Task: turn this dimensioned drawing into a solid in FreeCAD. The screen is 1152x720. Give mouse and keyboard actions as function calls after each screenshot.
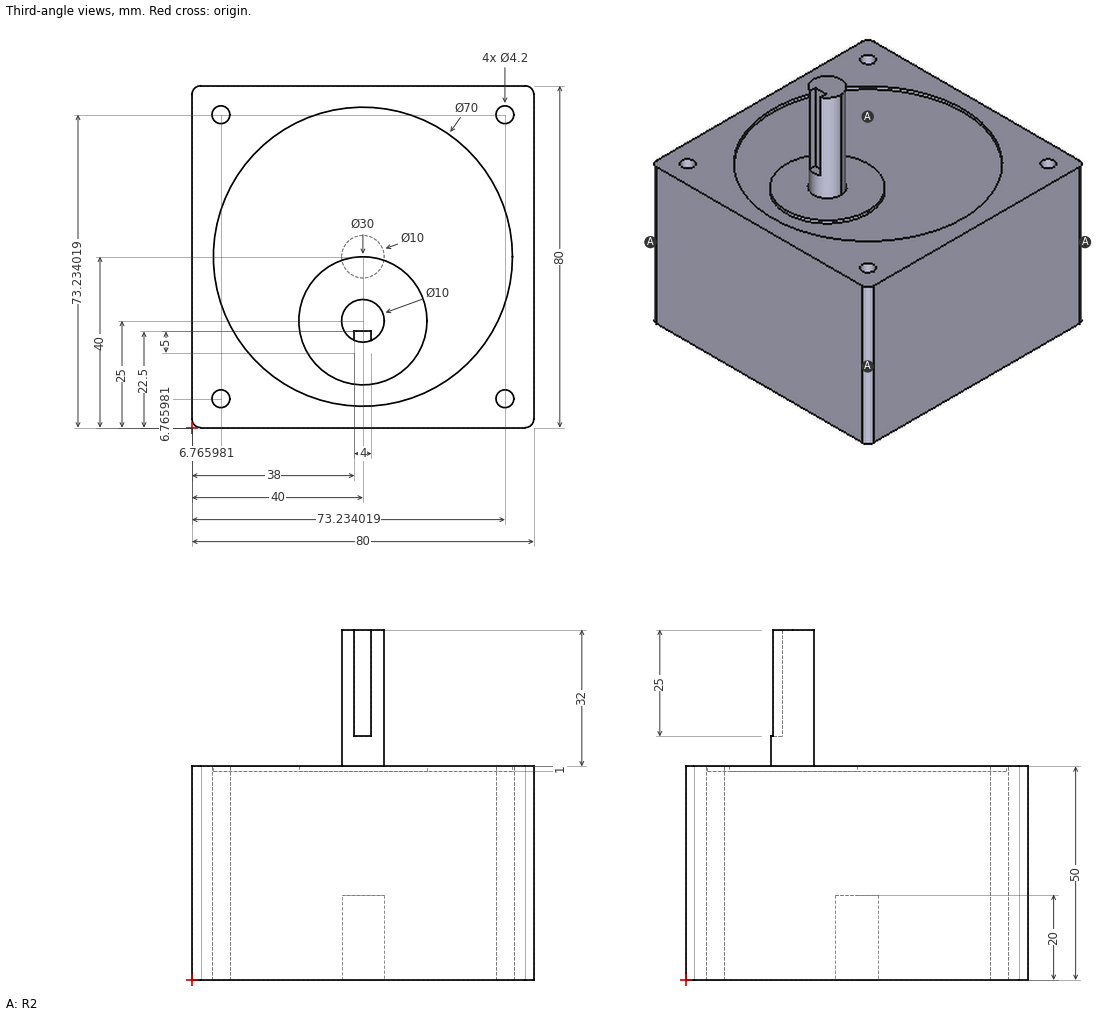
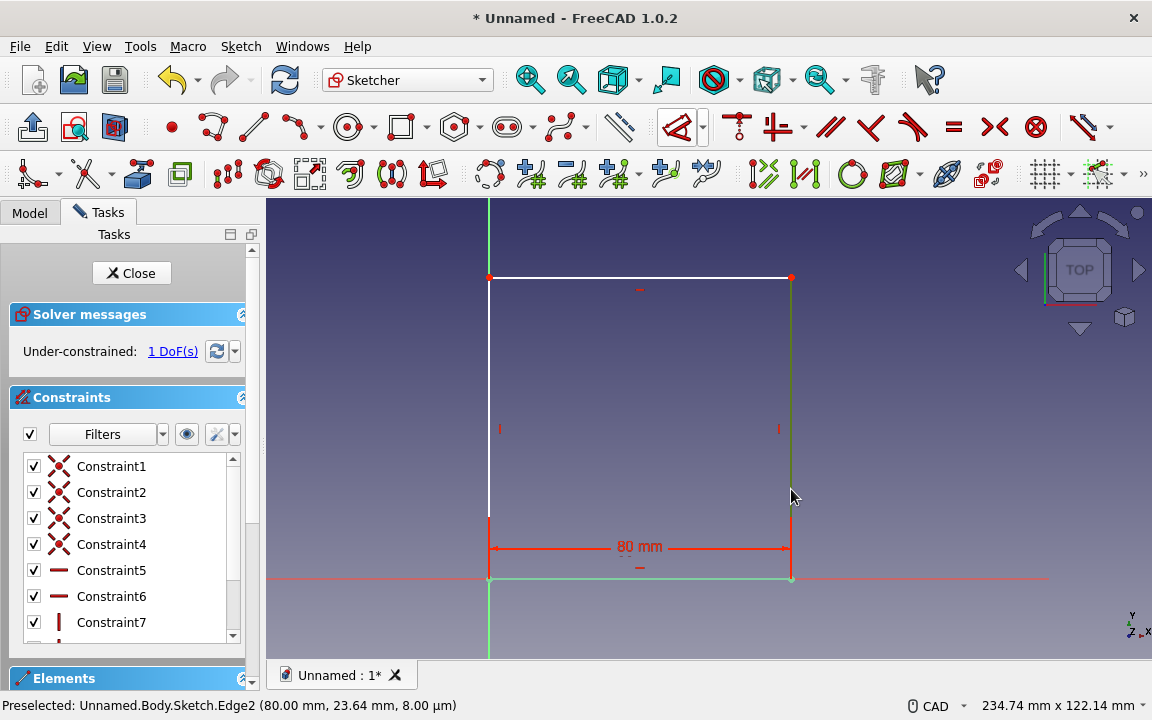
click(702, 128)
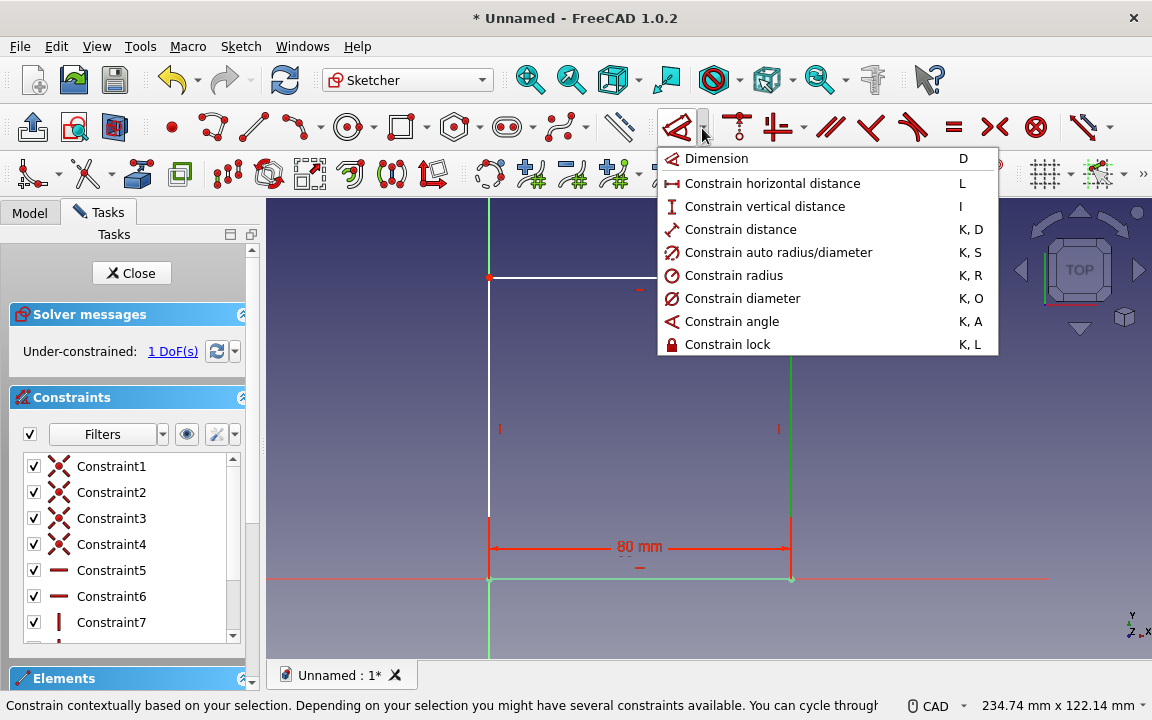
click(828, 206)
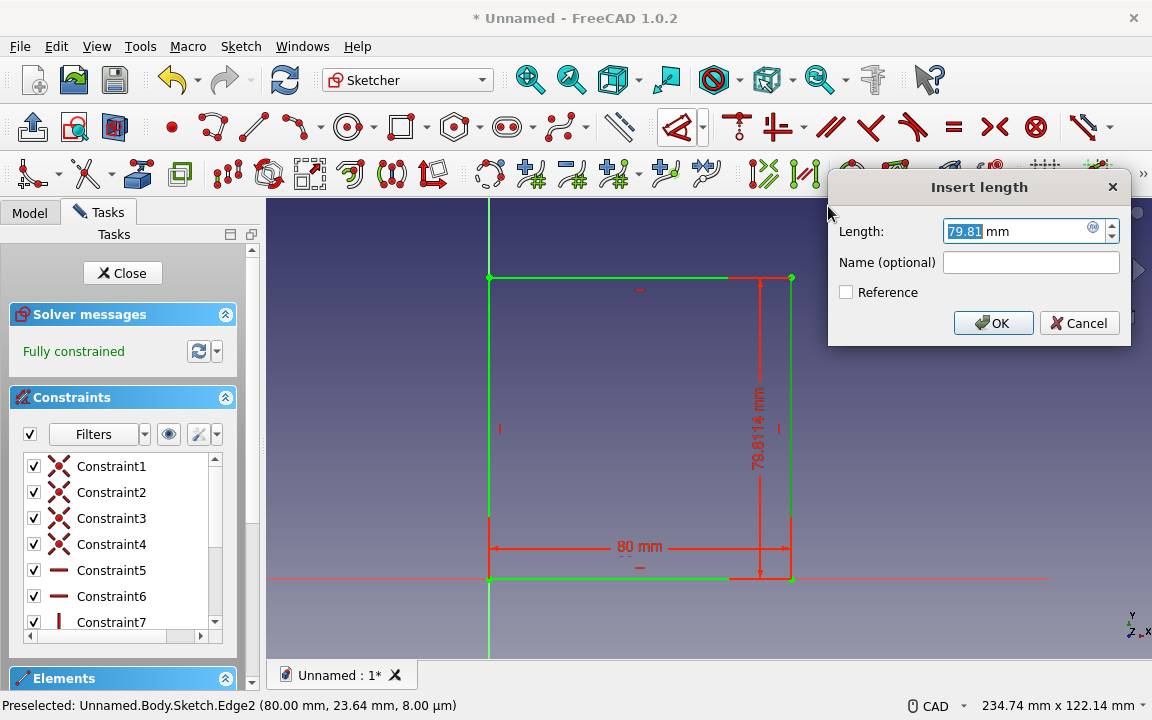
text(80)
key(Return)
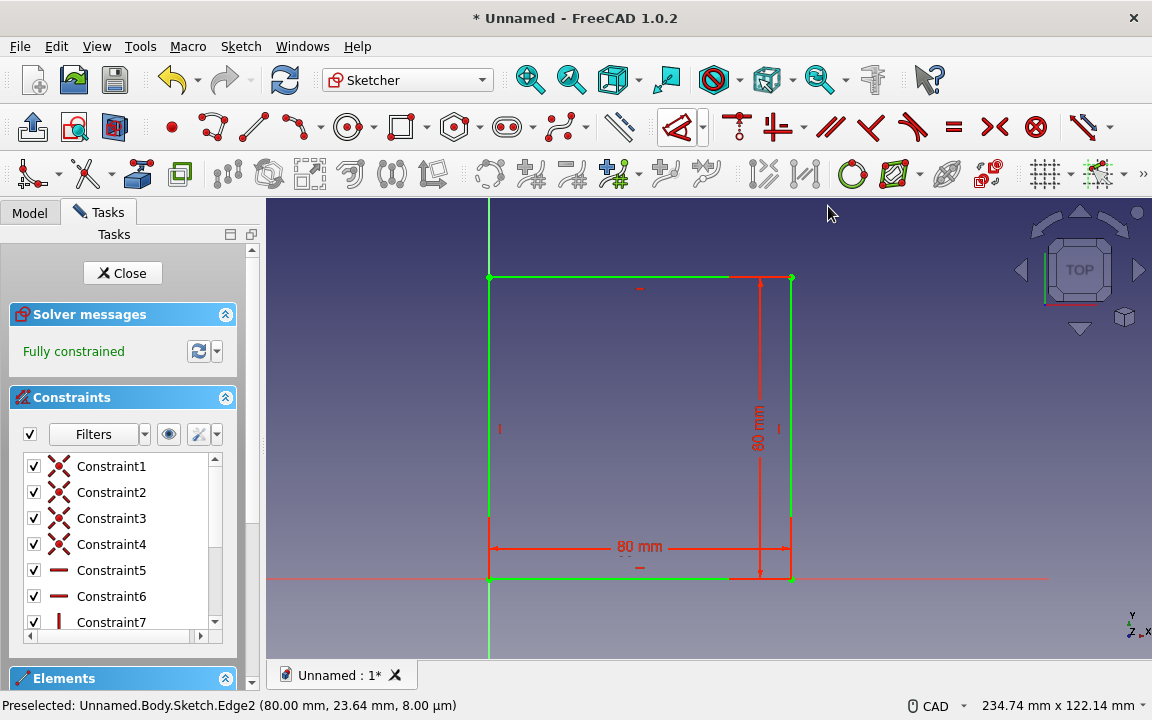
click(123, 273)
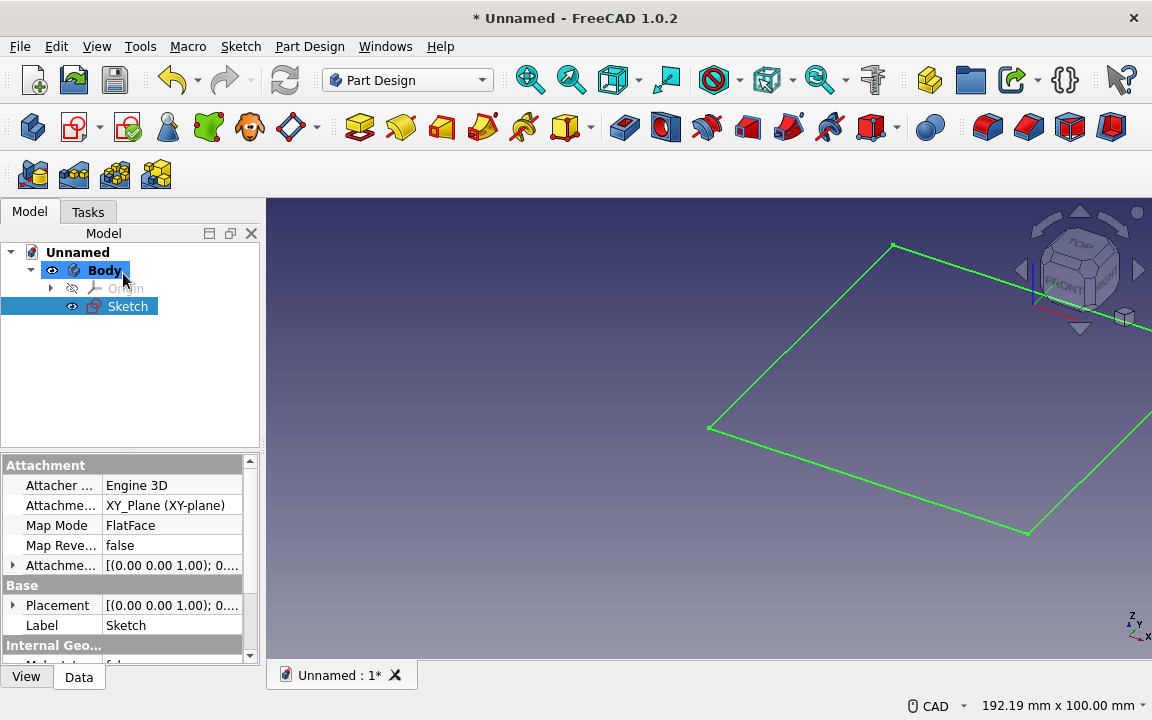
click(360, 128)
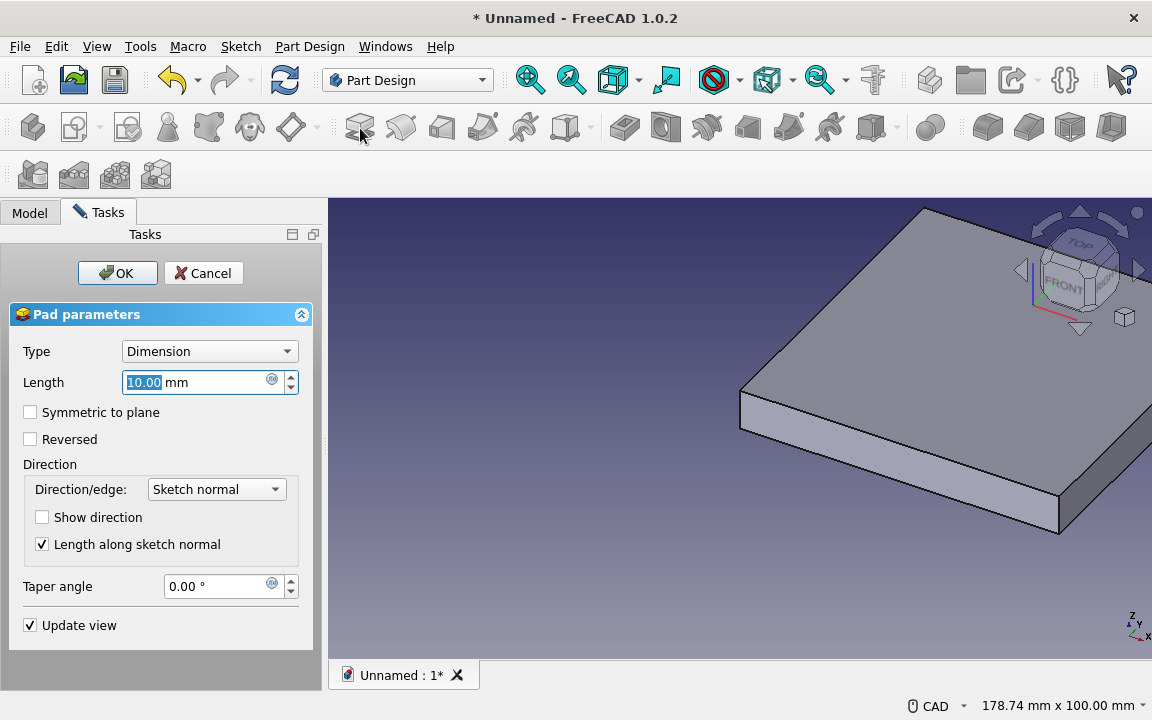
text(50)
key(Tab)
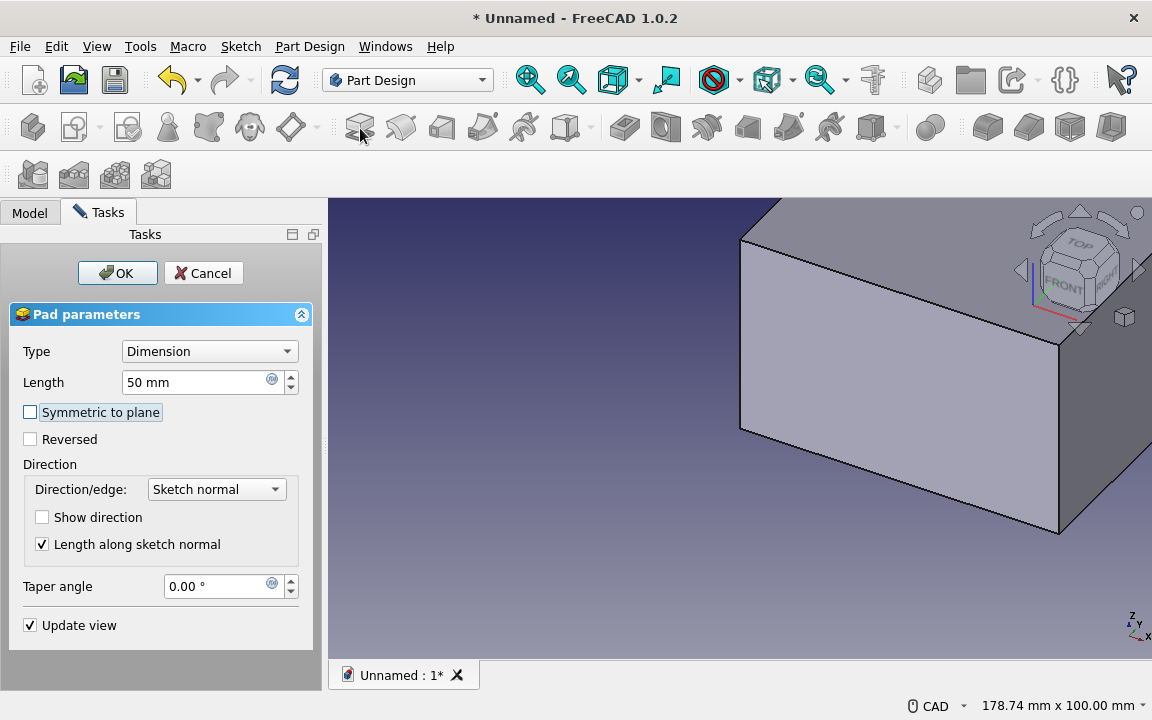
click(118, 273)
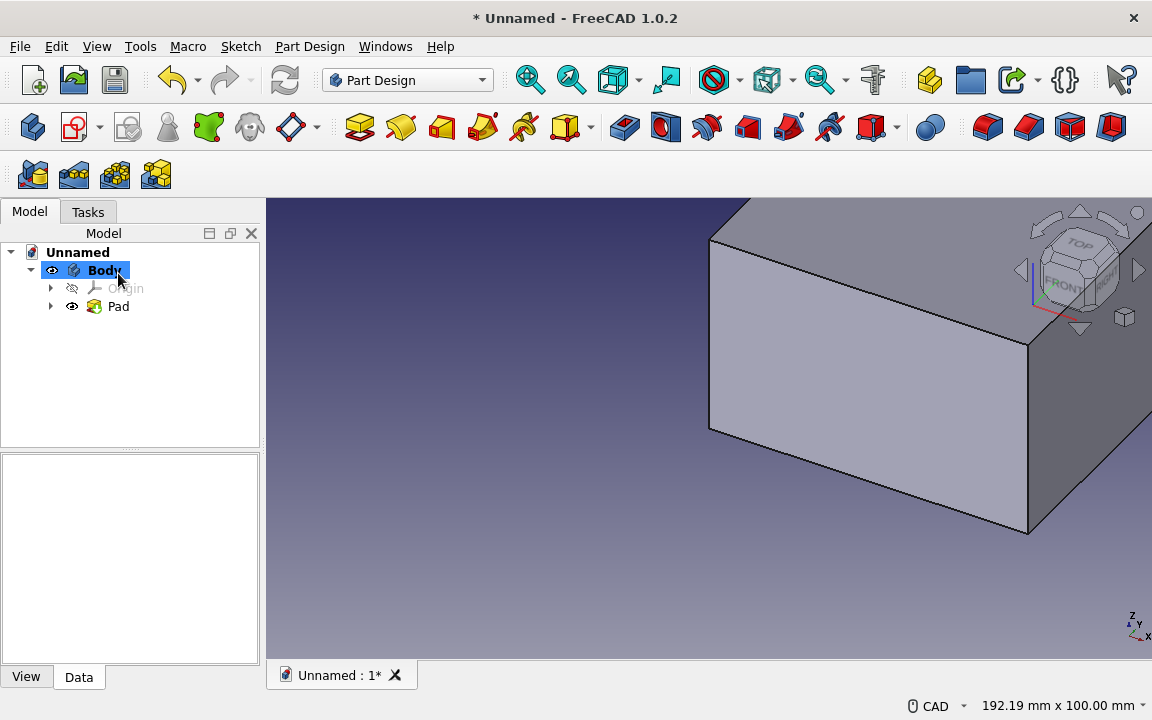
click(531, 80)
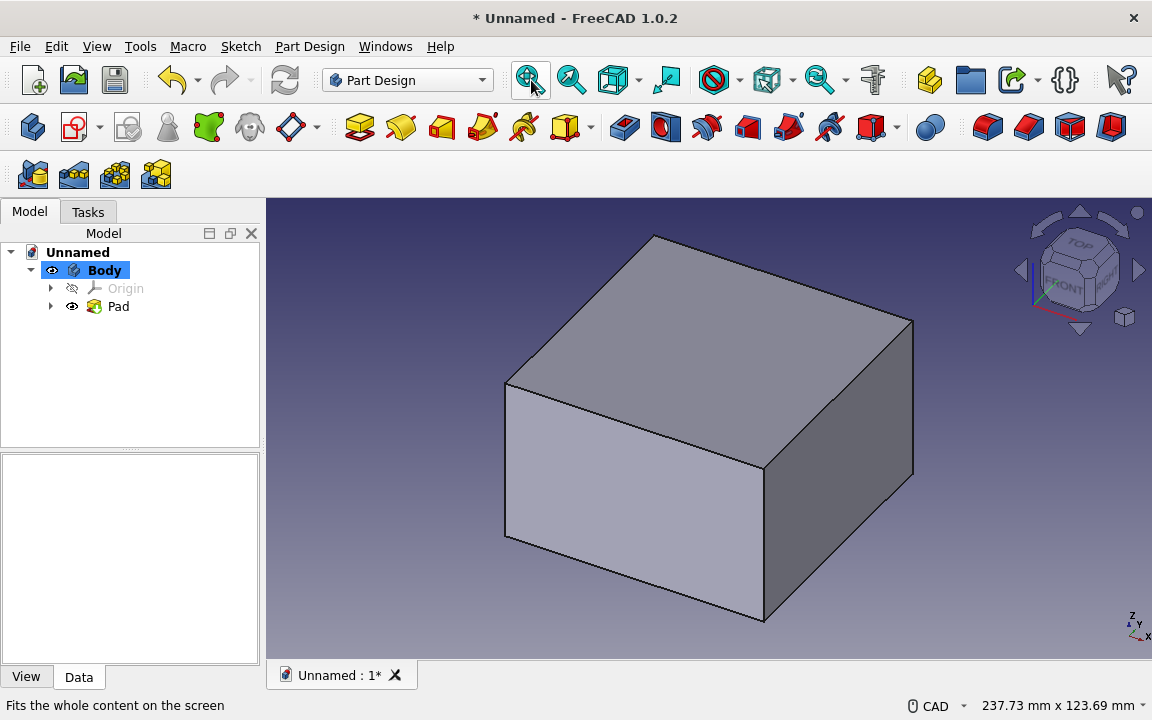
click(709, 351)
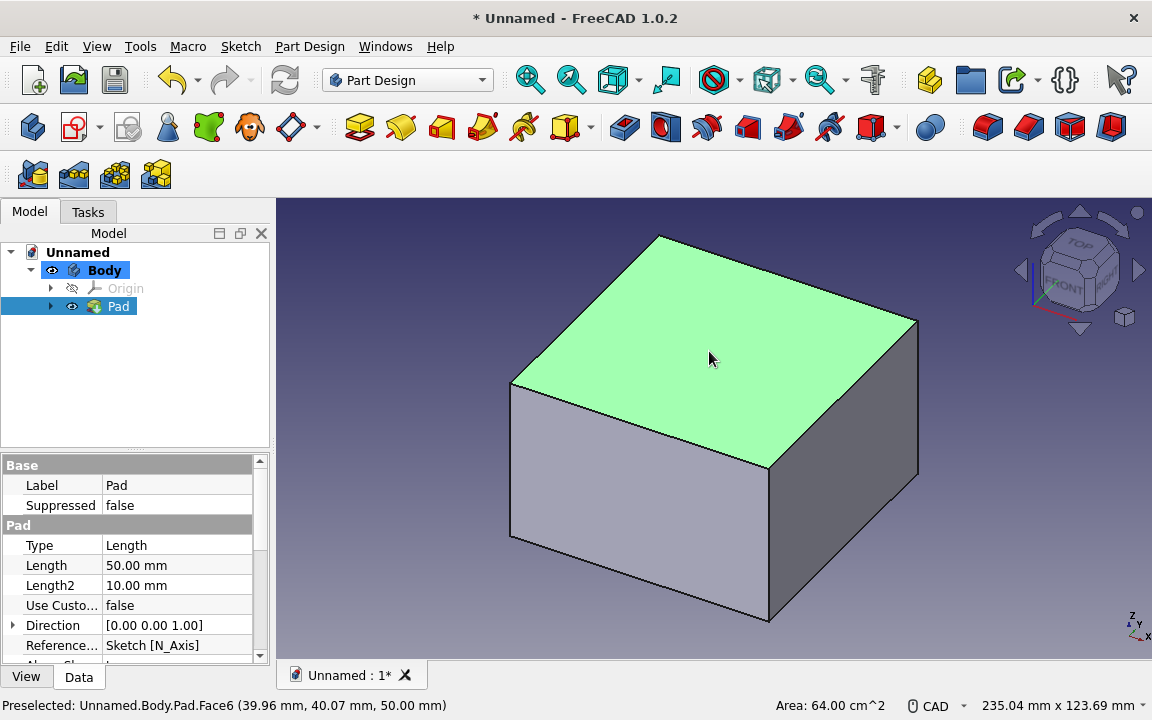
click(74, 128)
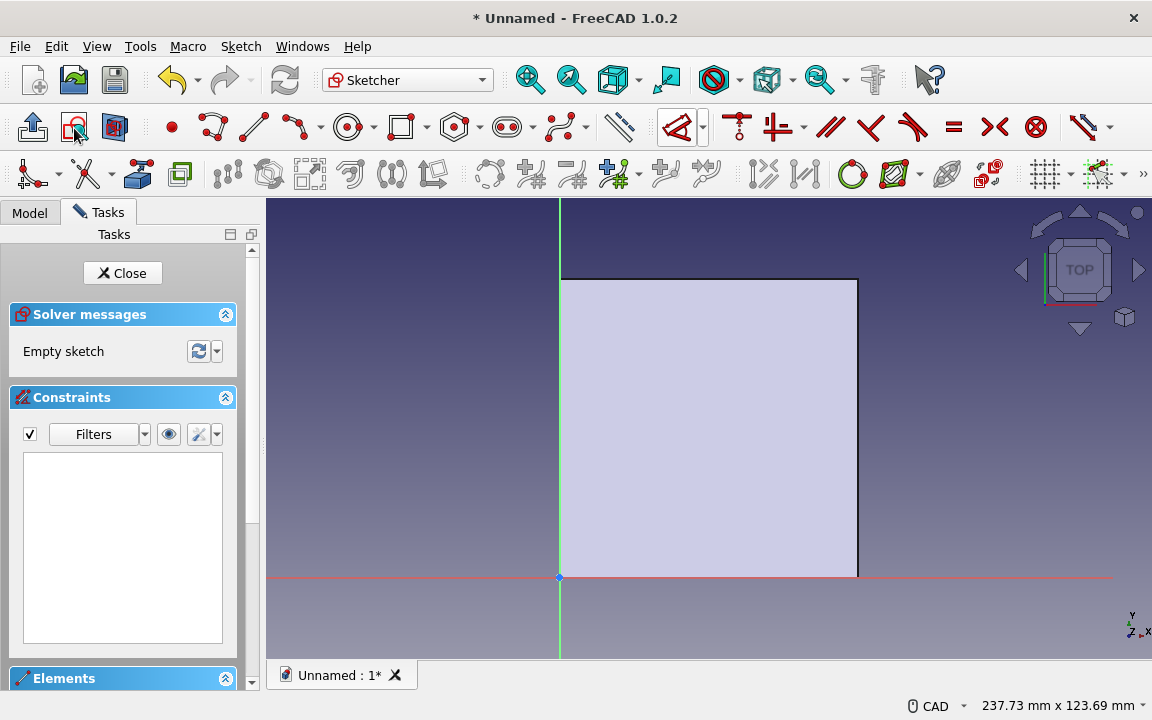
click(348, 128)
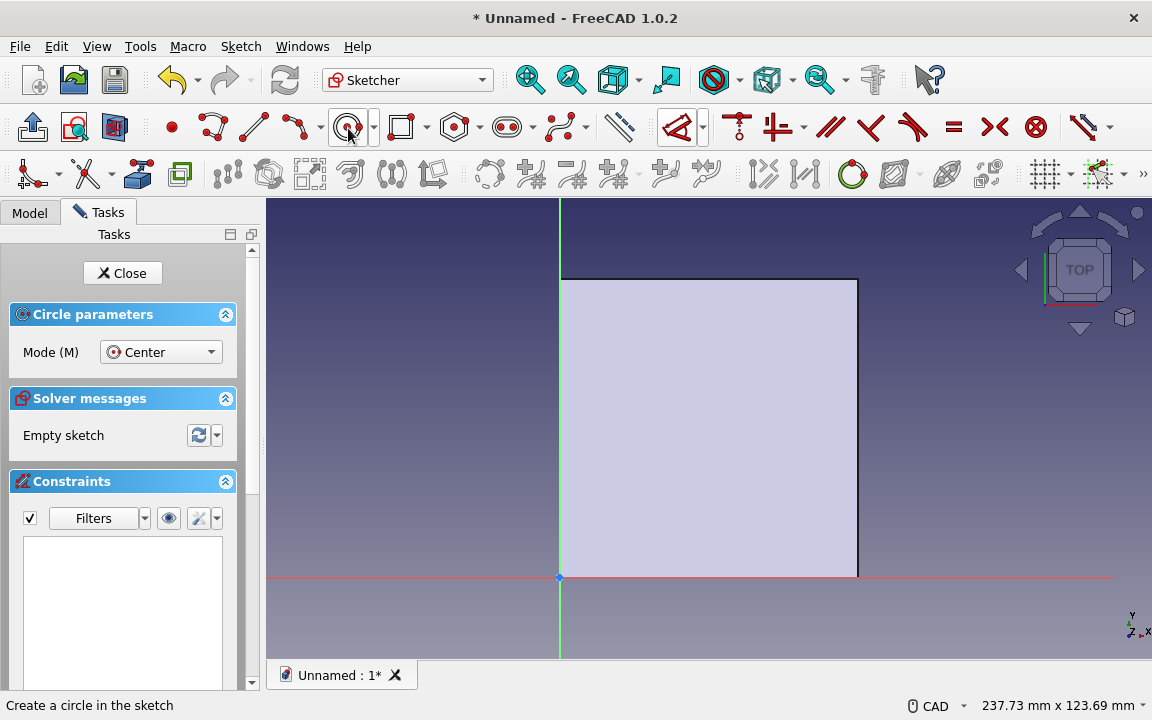
click(709, 428)
click(801, 336)
key(Escape)